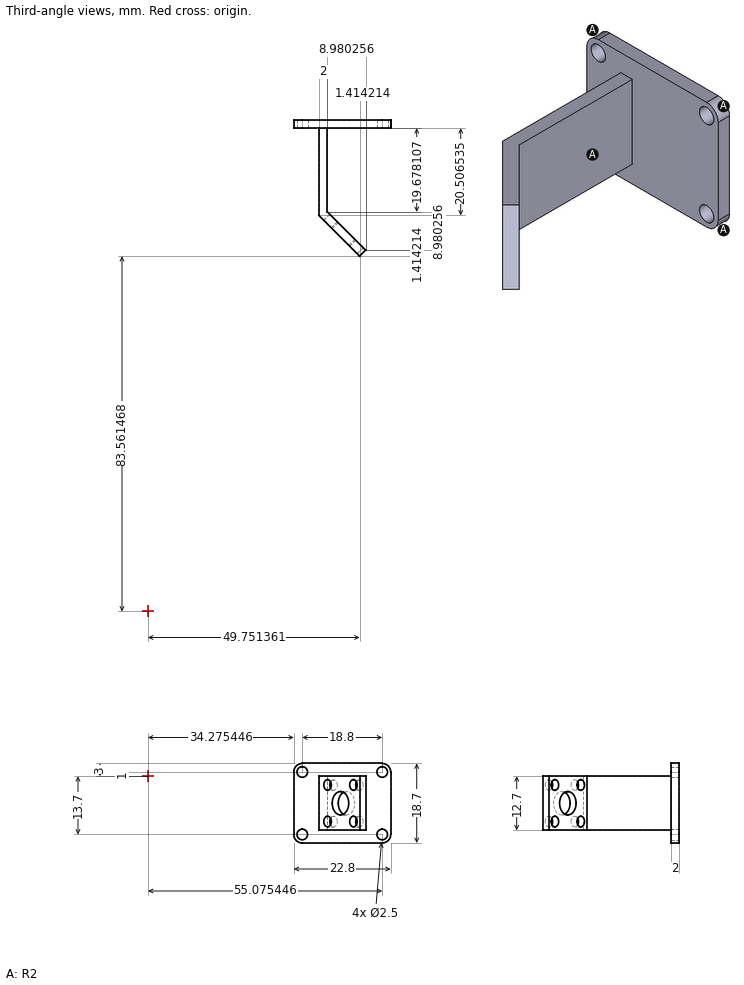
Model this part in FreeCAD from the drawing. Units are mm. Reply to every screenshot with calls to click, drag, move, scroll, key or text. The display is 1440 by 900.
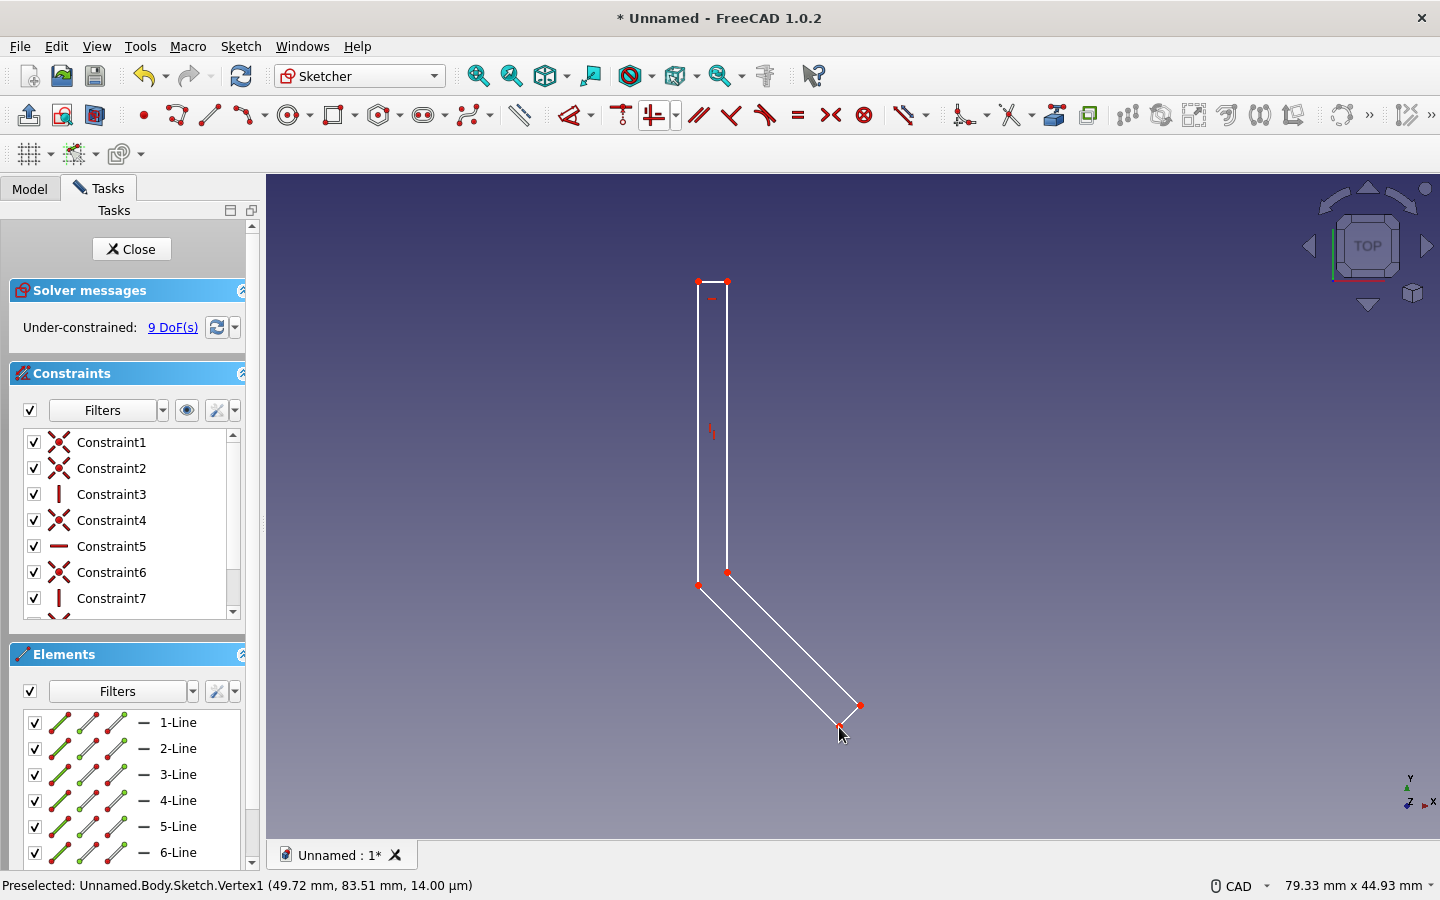
key(d)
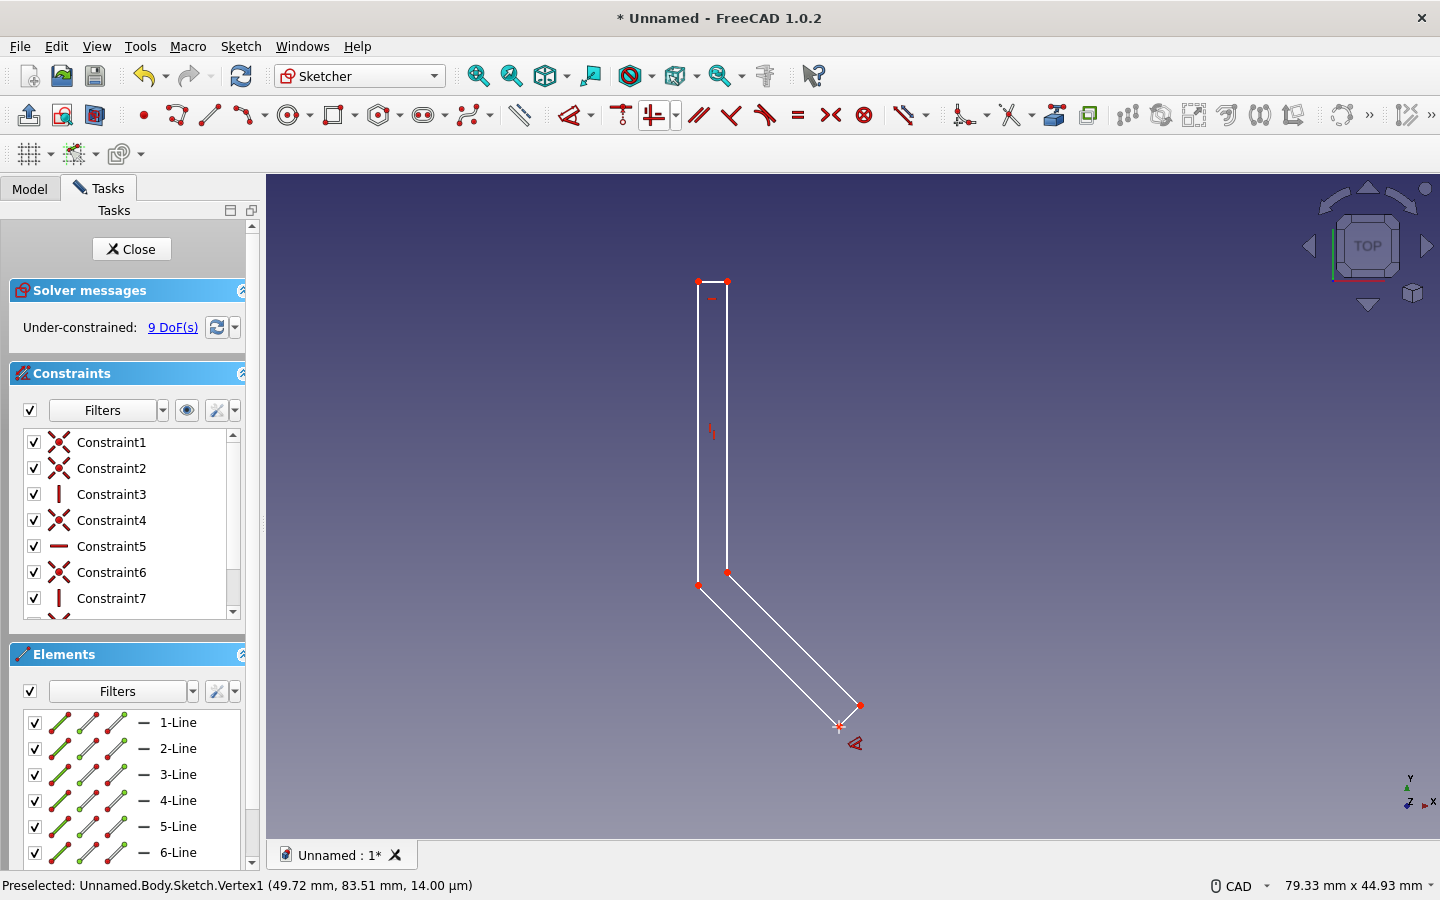
scroll(715, 282, up, 2)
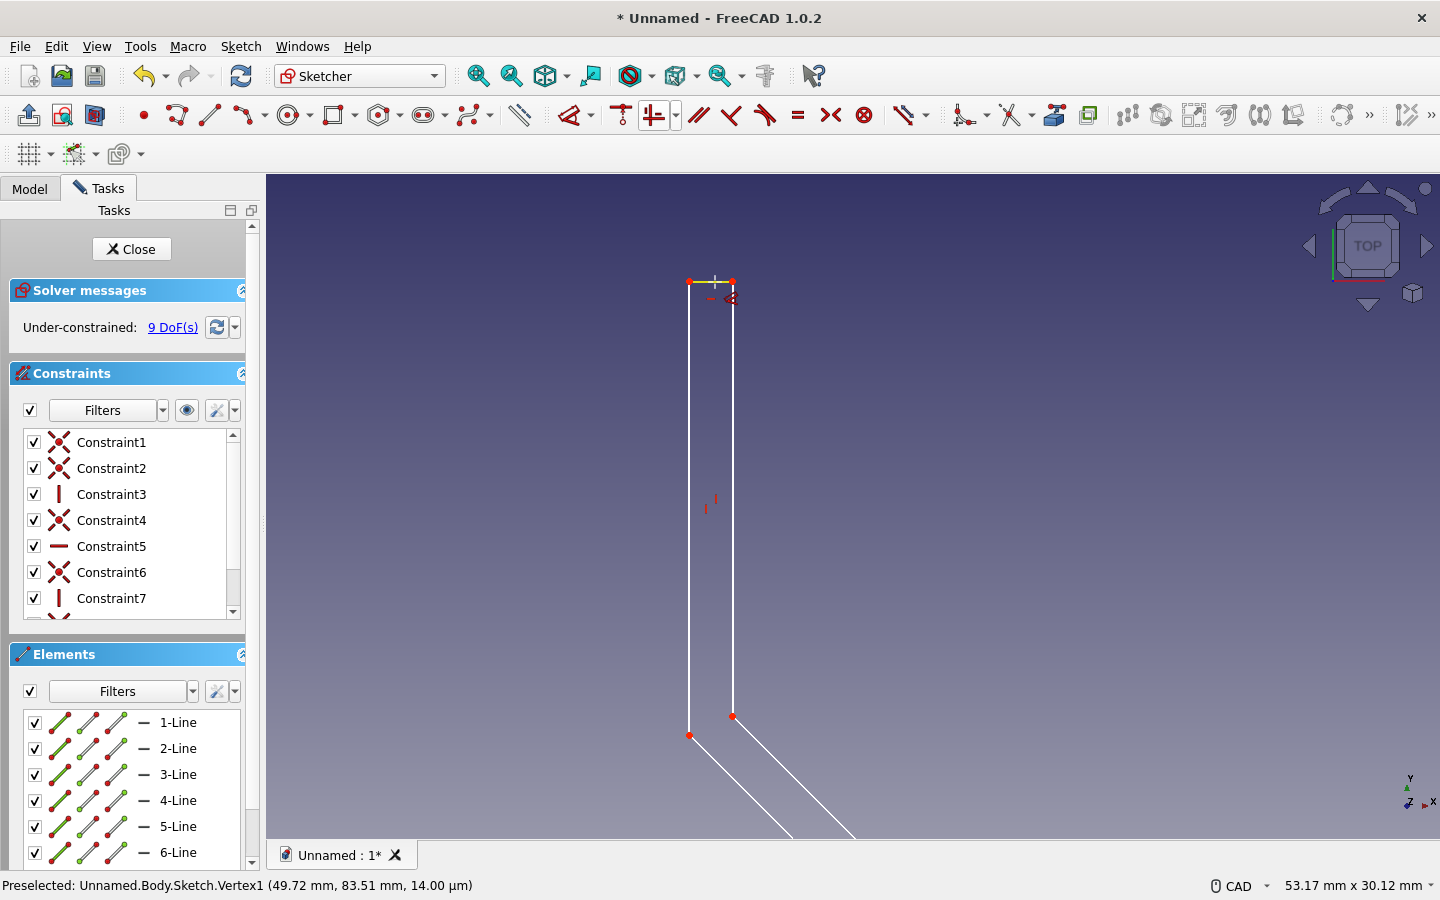
click(715, 282)
click(711, 248)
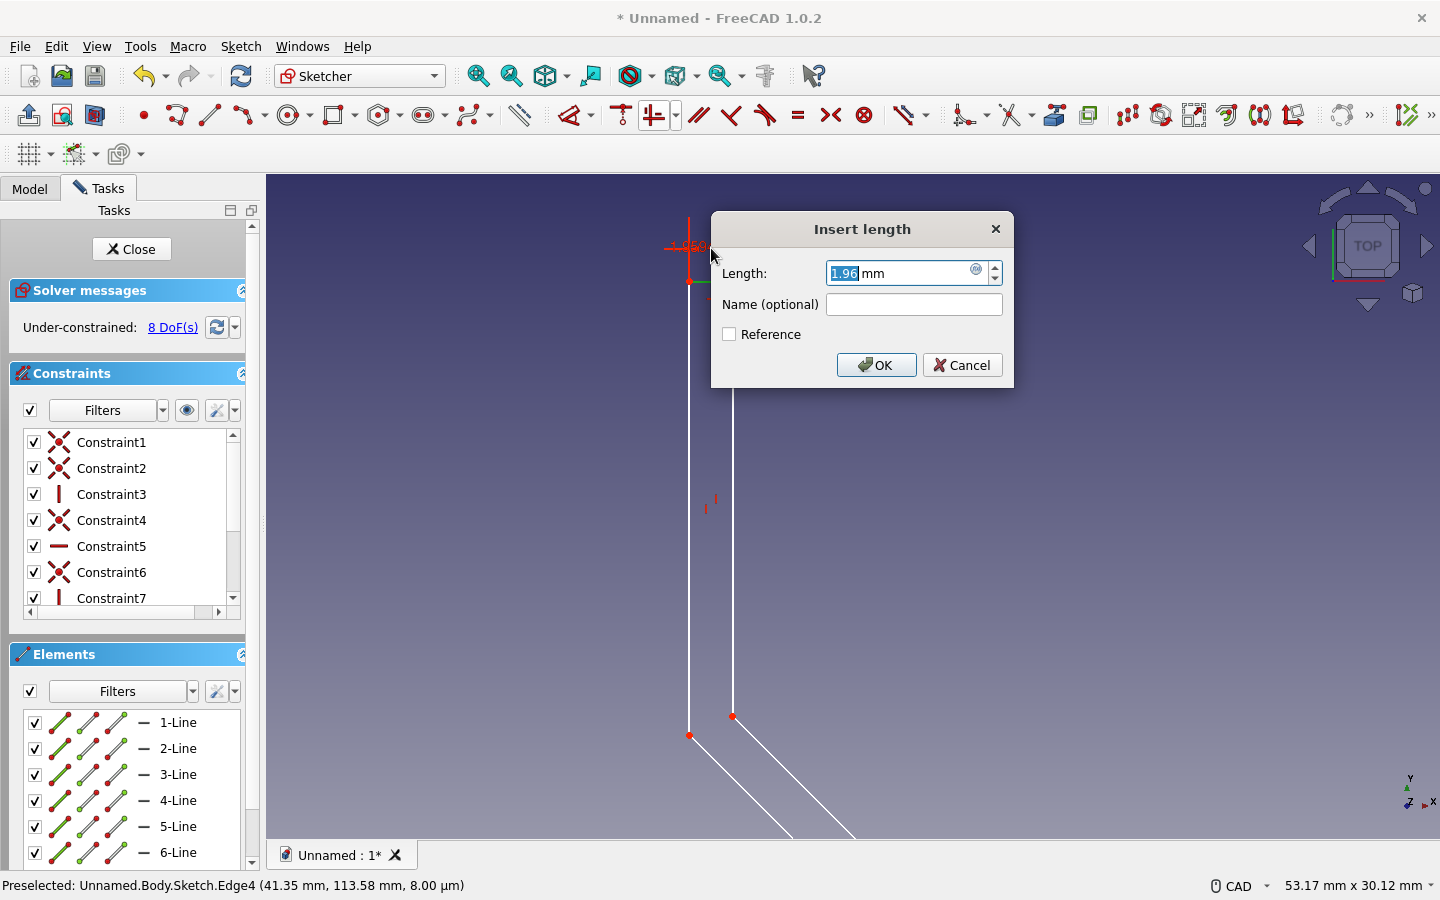
text(2)
key(Return)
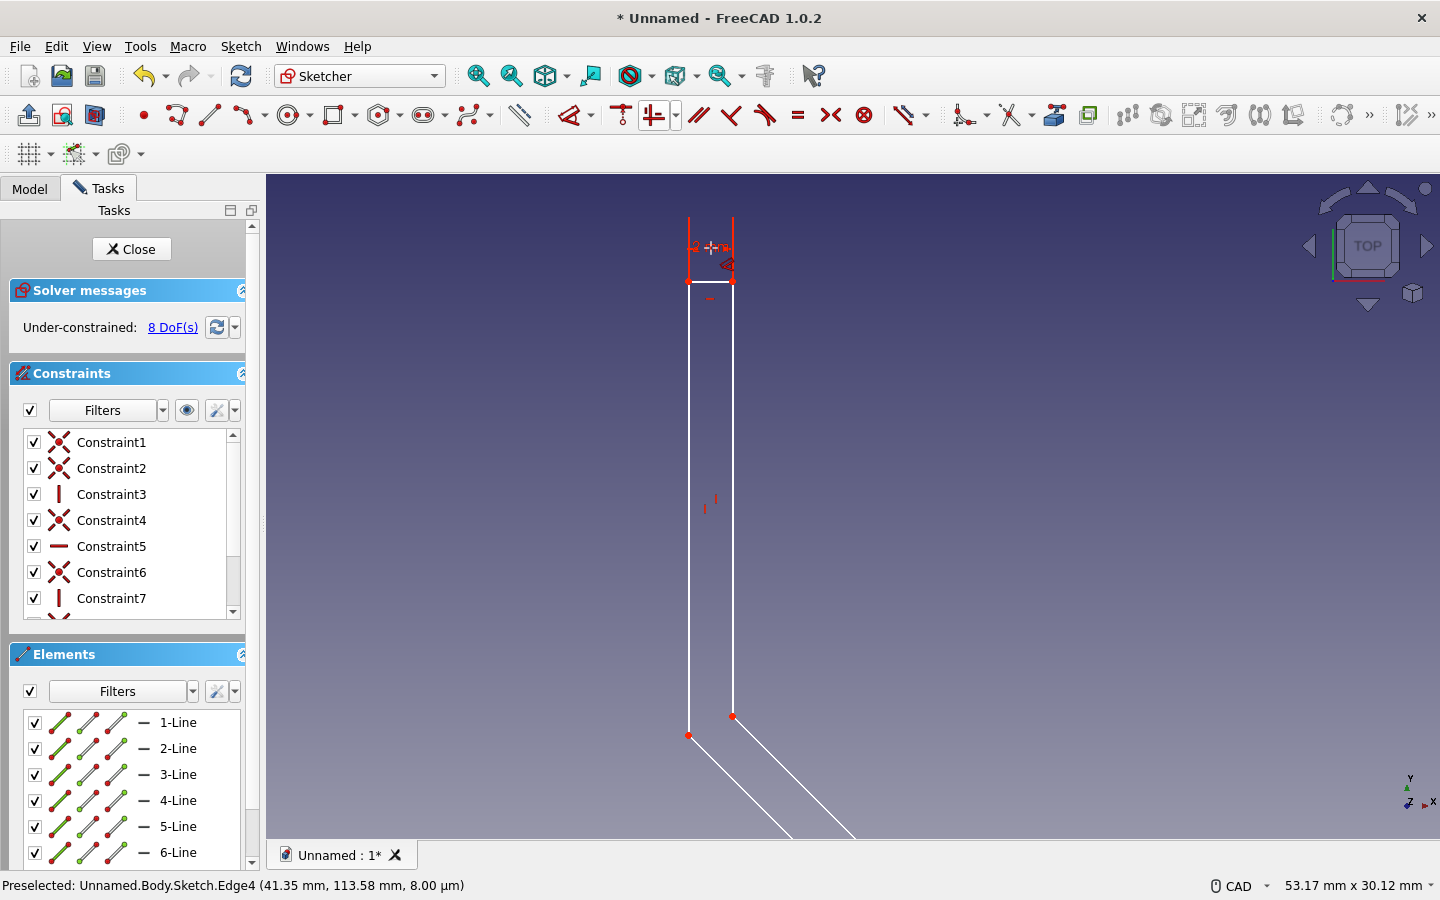
click(733, 586)
click(767, 499)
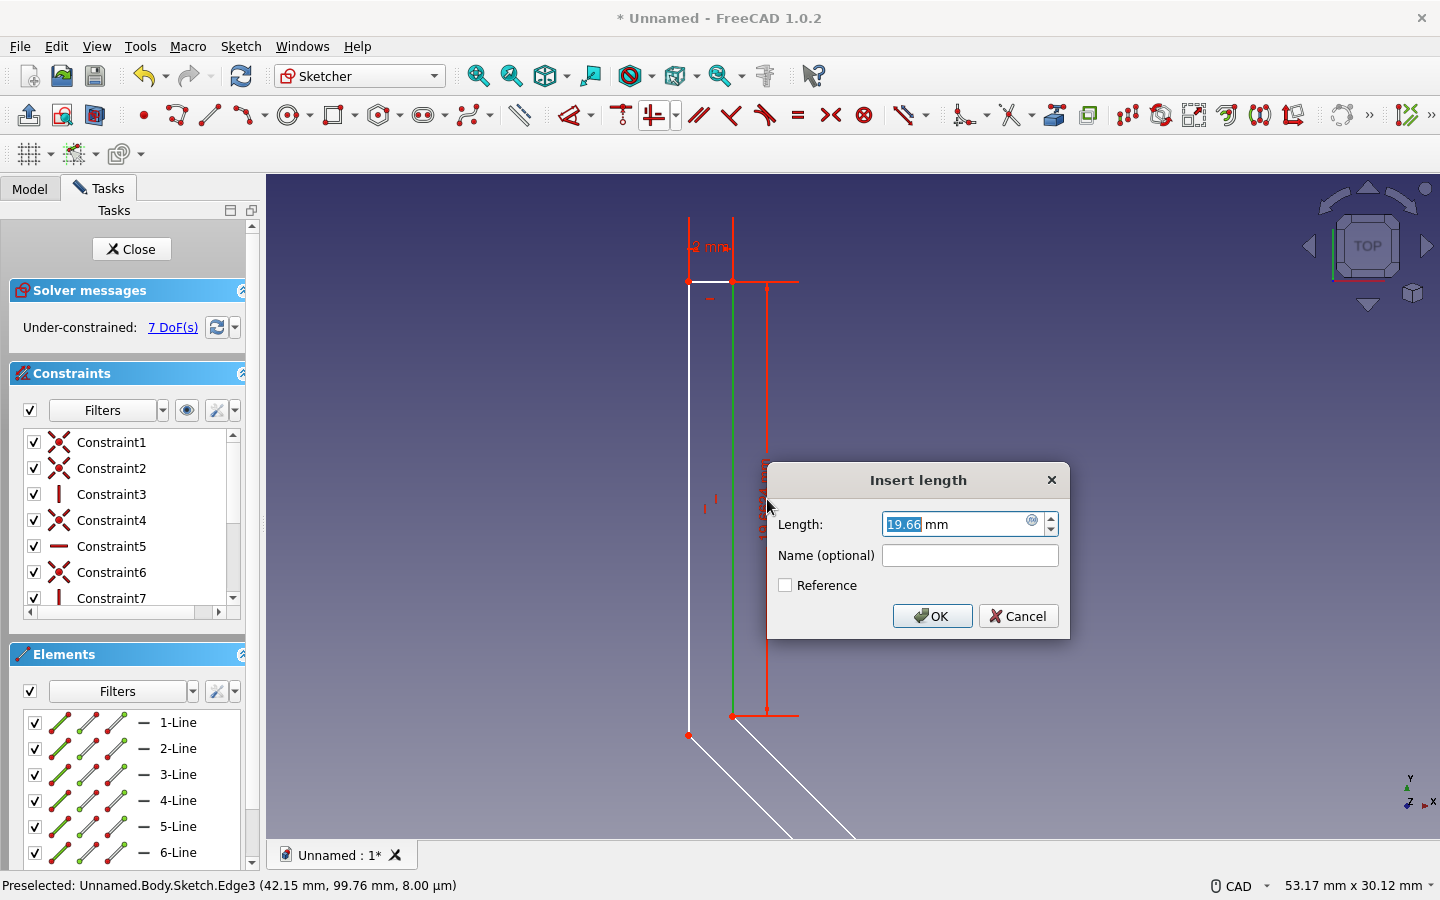
text(19.678107)
key(Return)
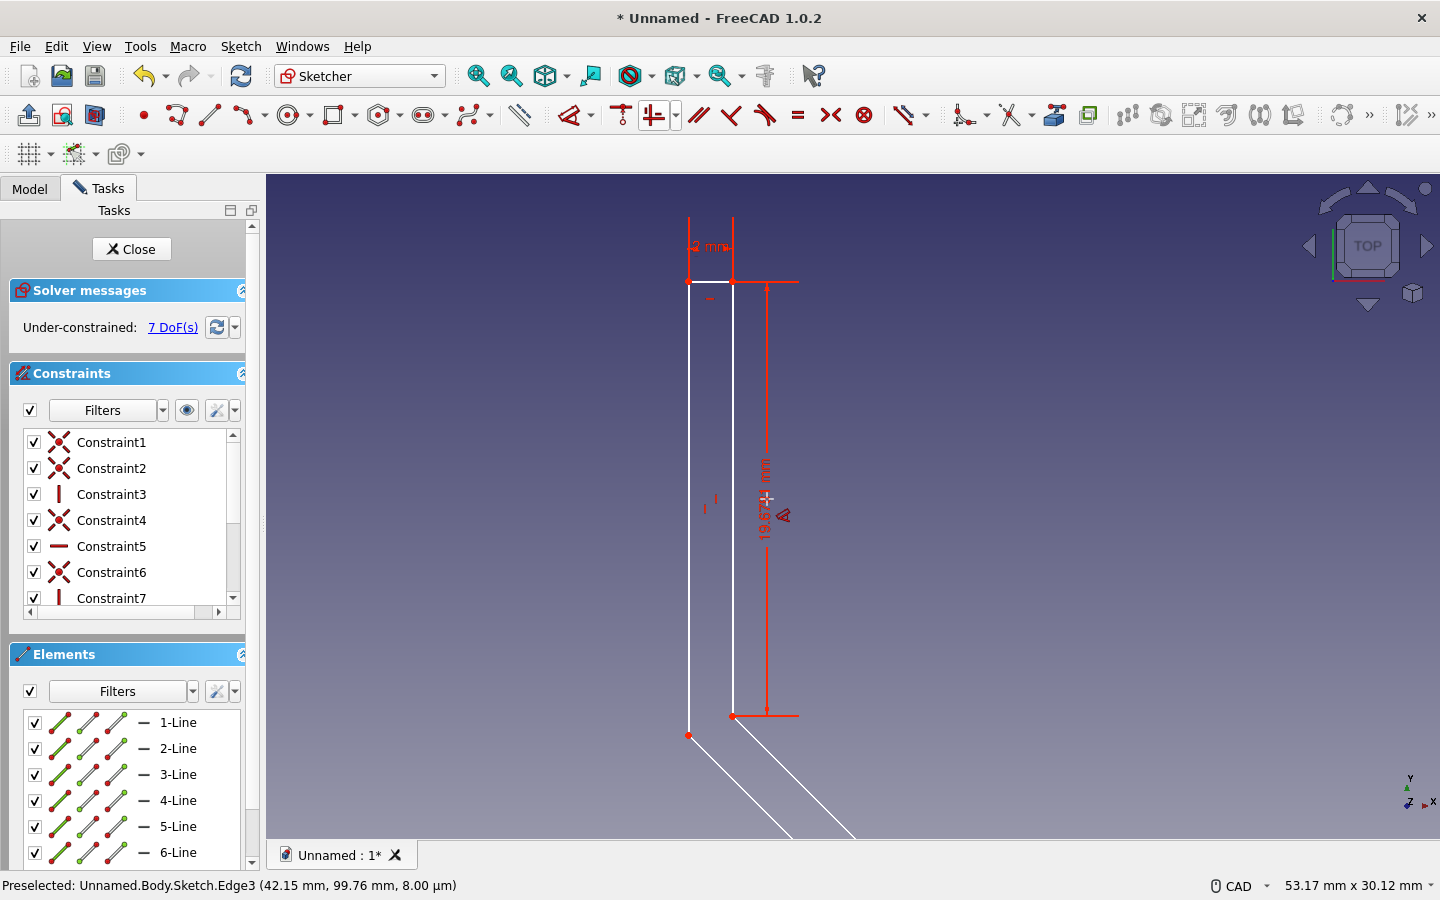
click(689, 418)
click(655, 509)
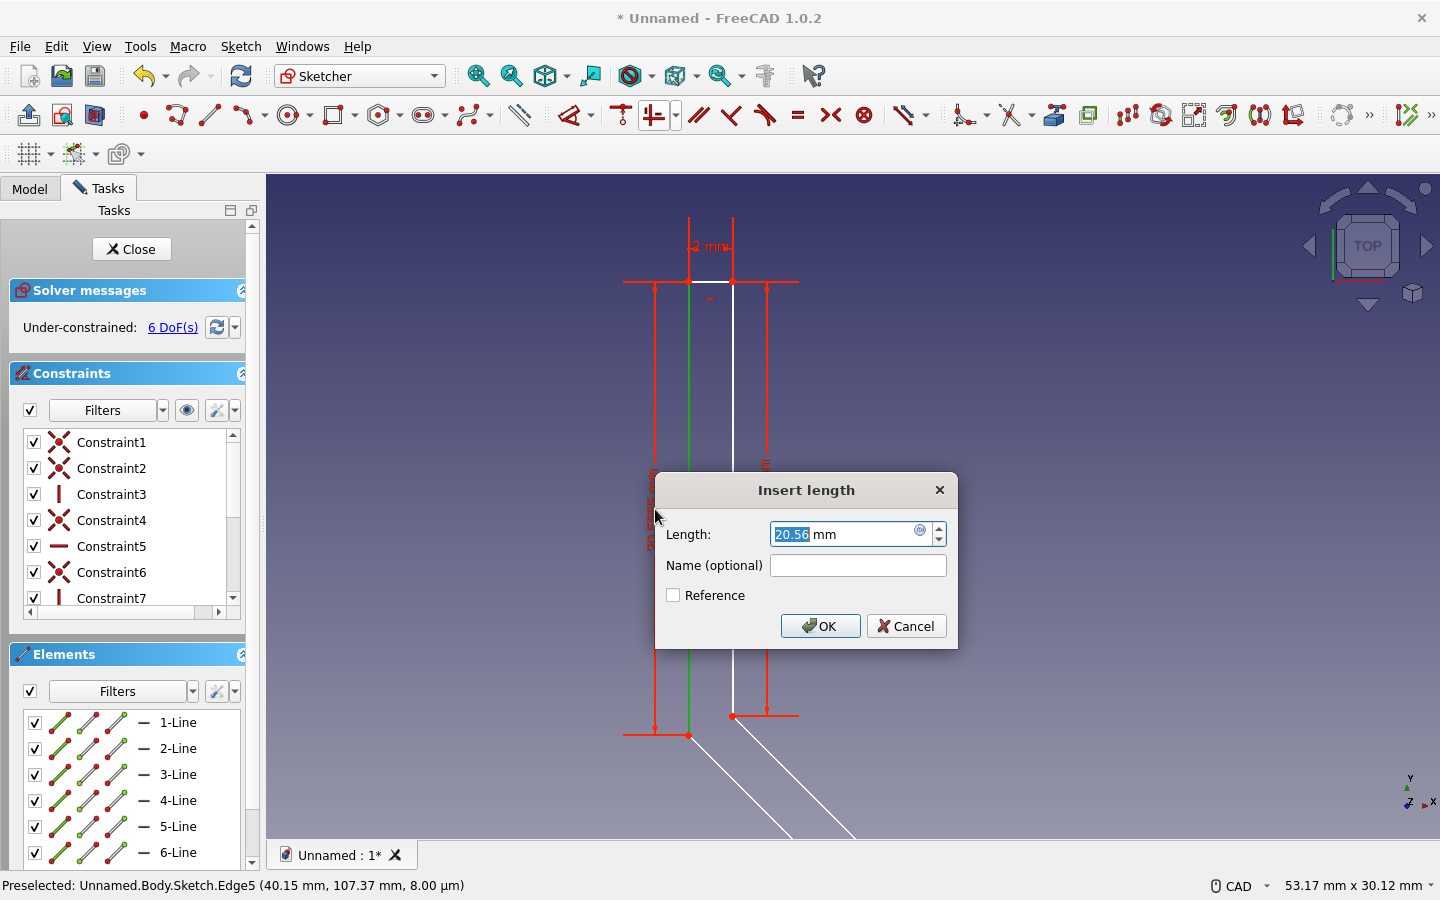
text(20.506535)
key(Return)